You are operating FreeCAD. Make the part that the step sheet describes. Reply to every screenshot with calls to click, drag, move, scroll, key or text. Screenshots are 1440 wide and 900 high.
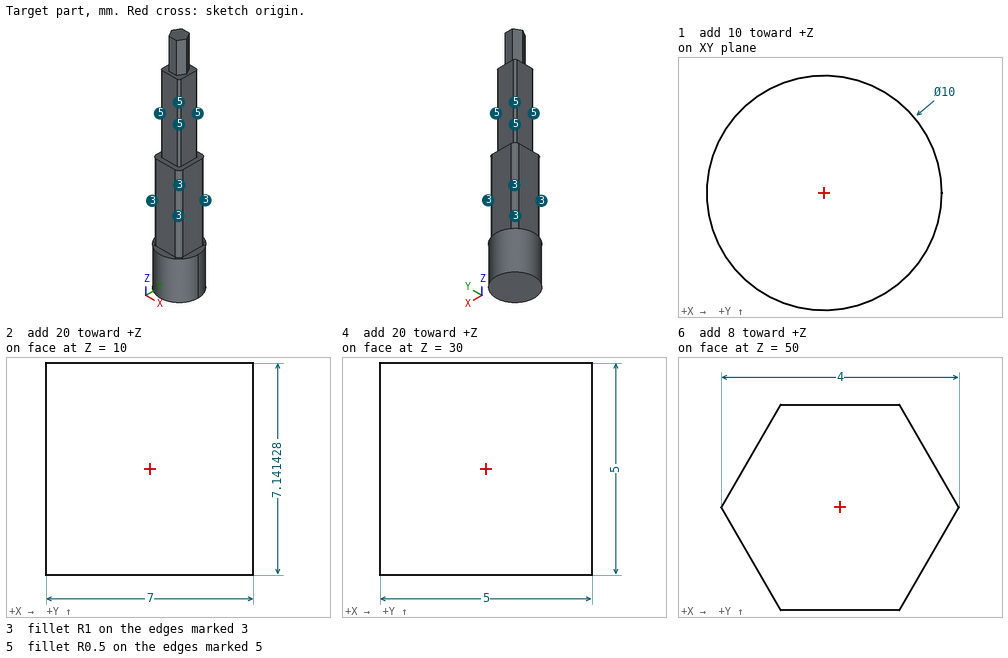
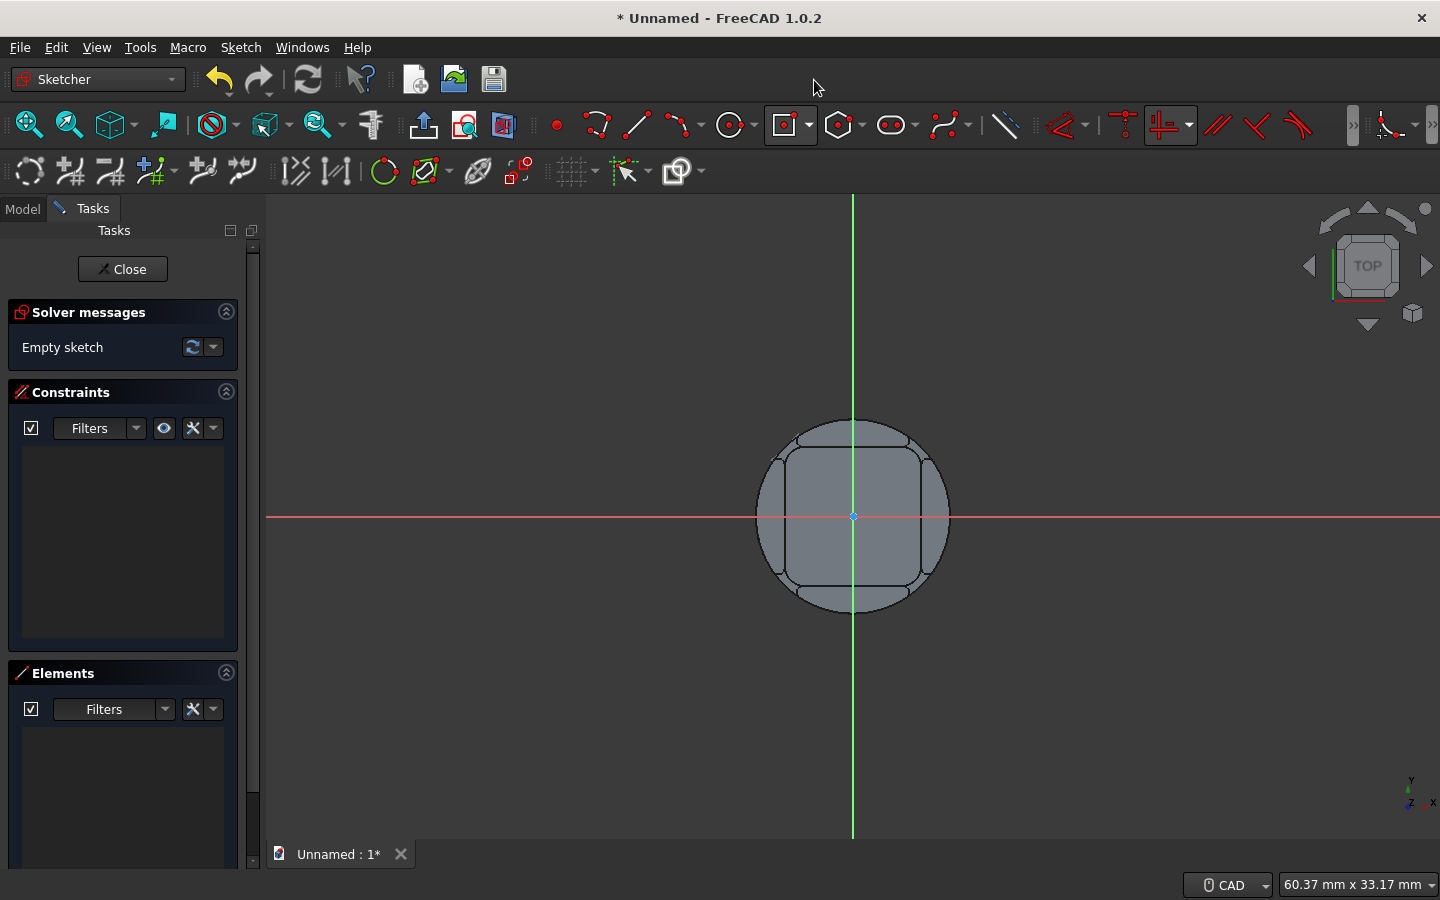
scroll(875, 516, up, 7)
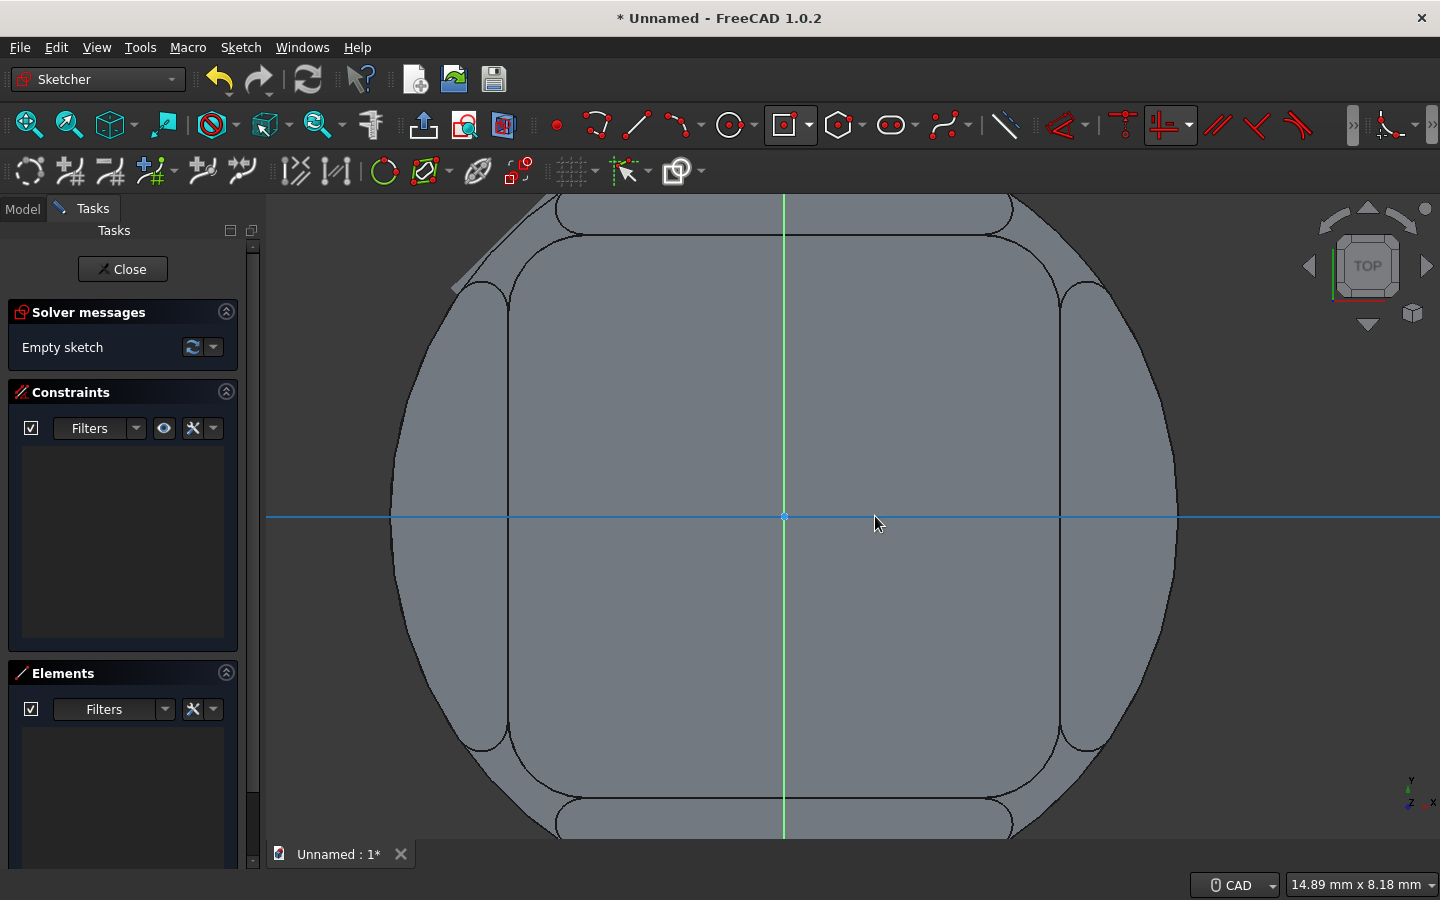
click(784, 126)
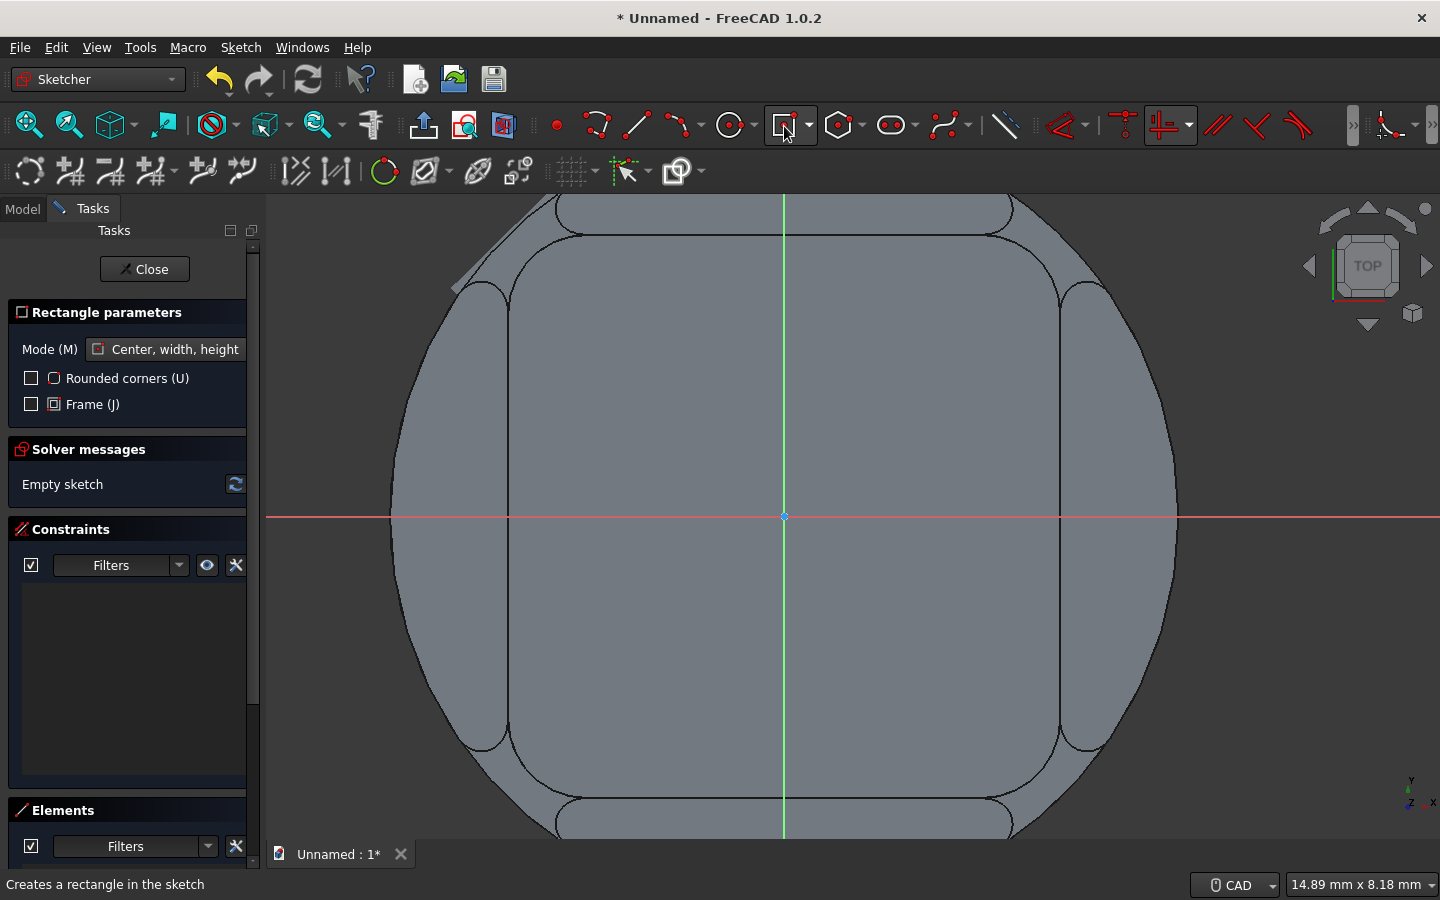
click(784, 516)
click(981, 319)
key(Escape)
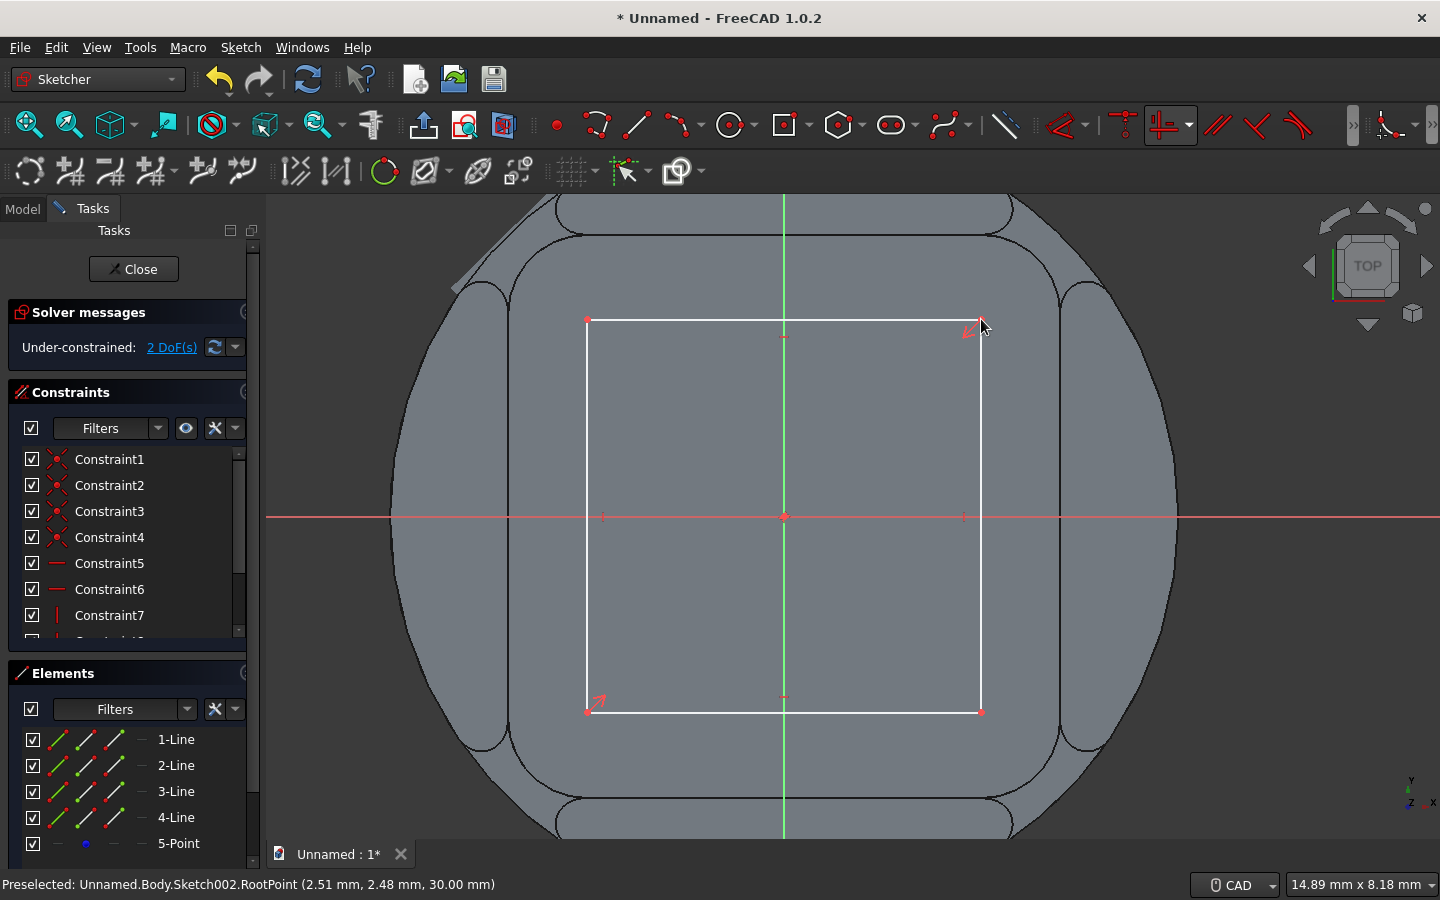
click(1060, 126)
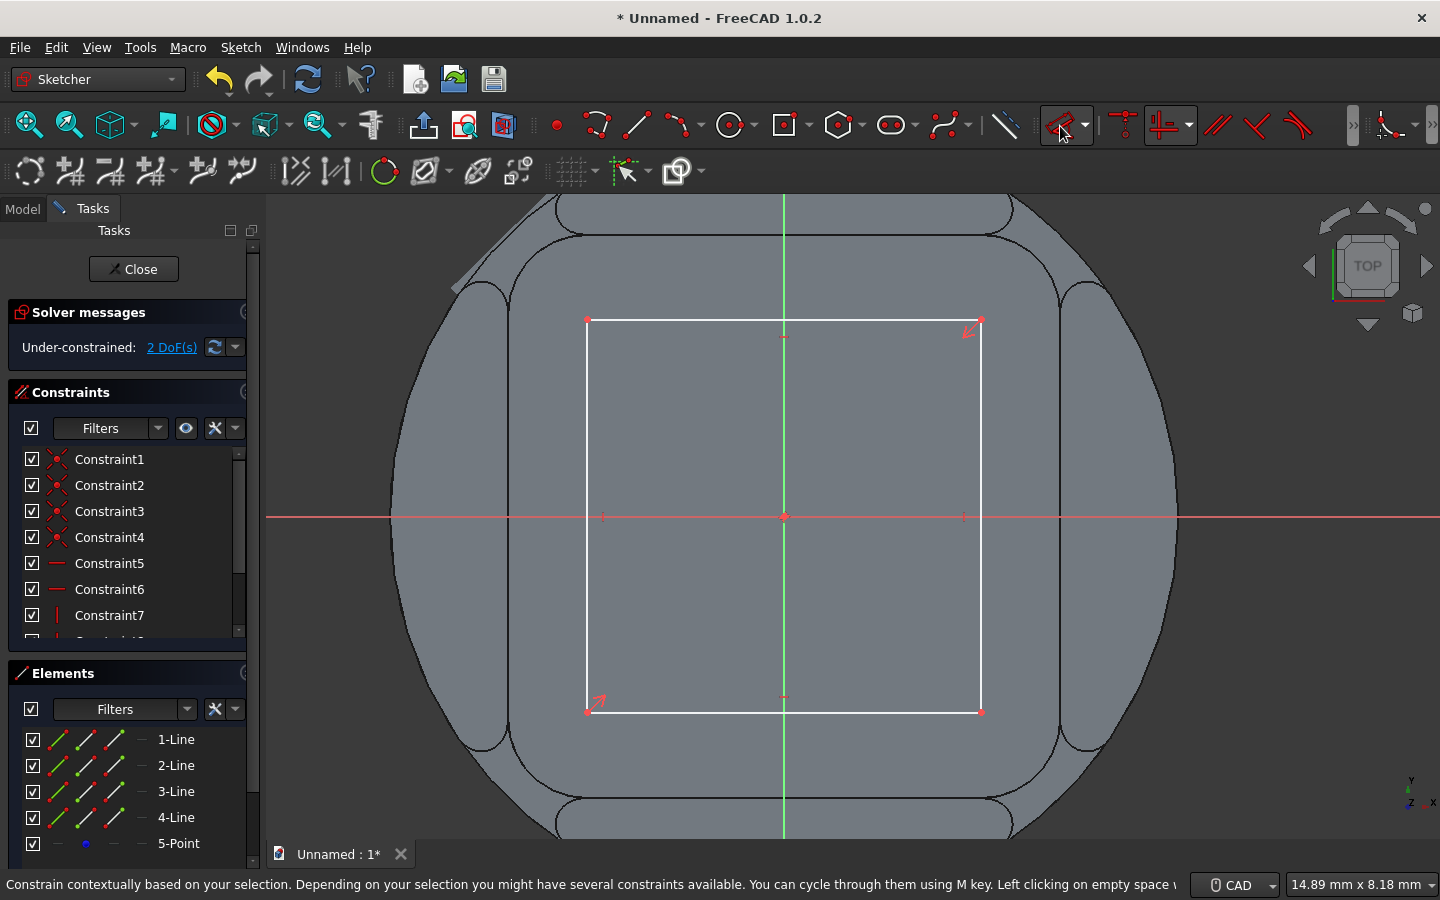
click(705, 713)
click(694, 747)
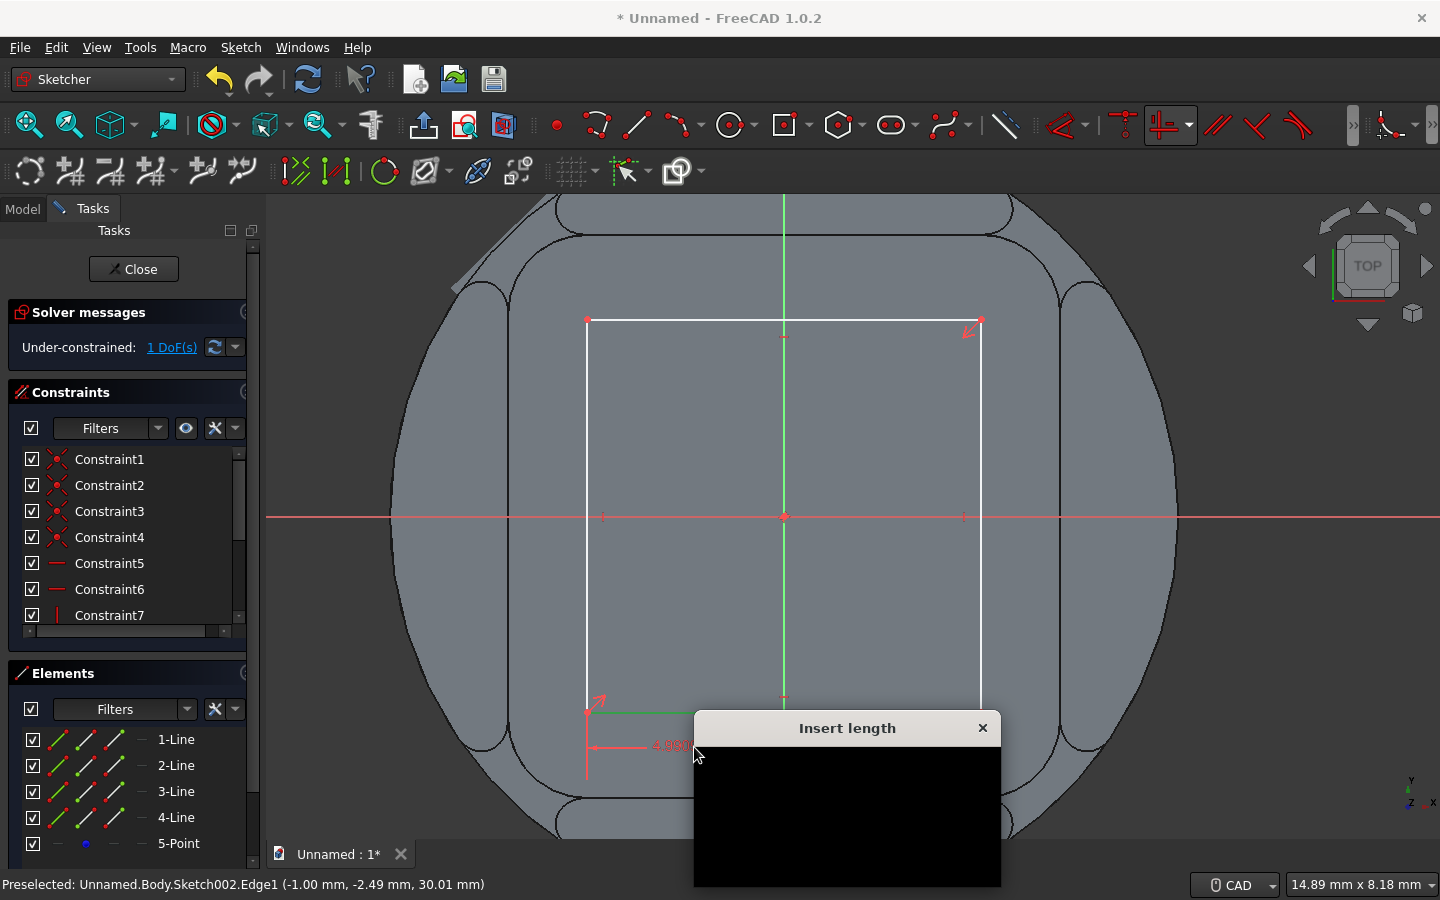
text(5)
key(Return)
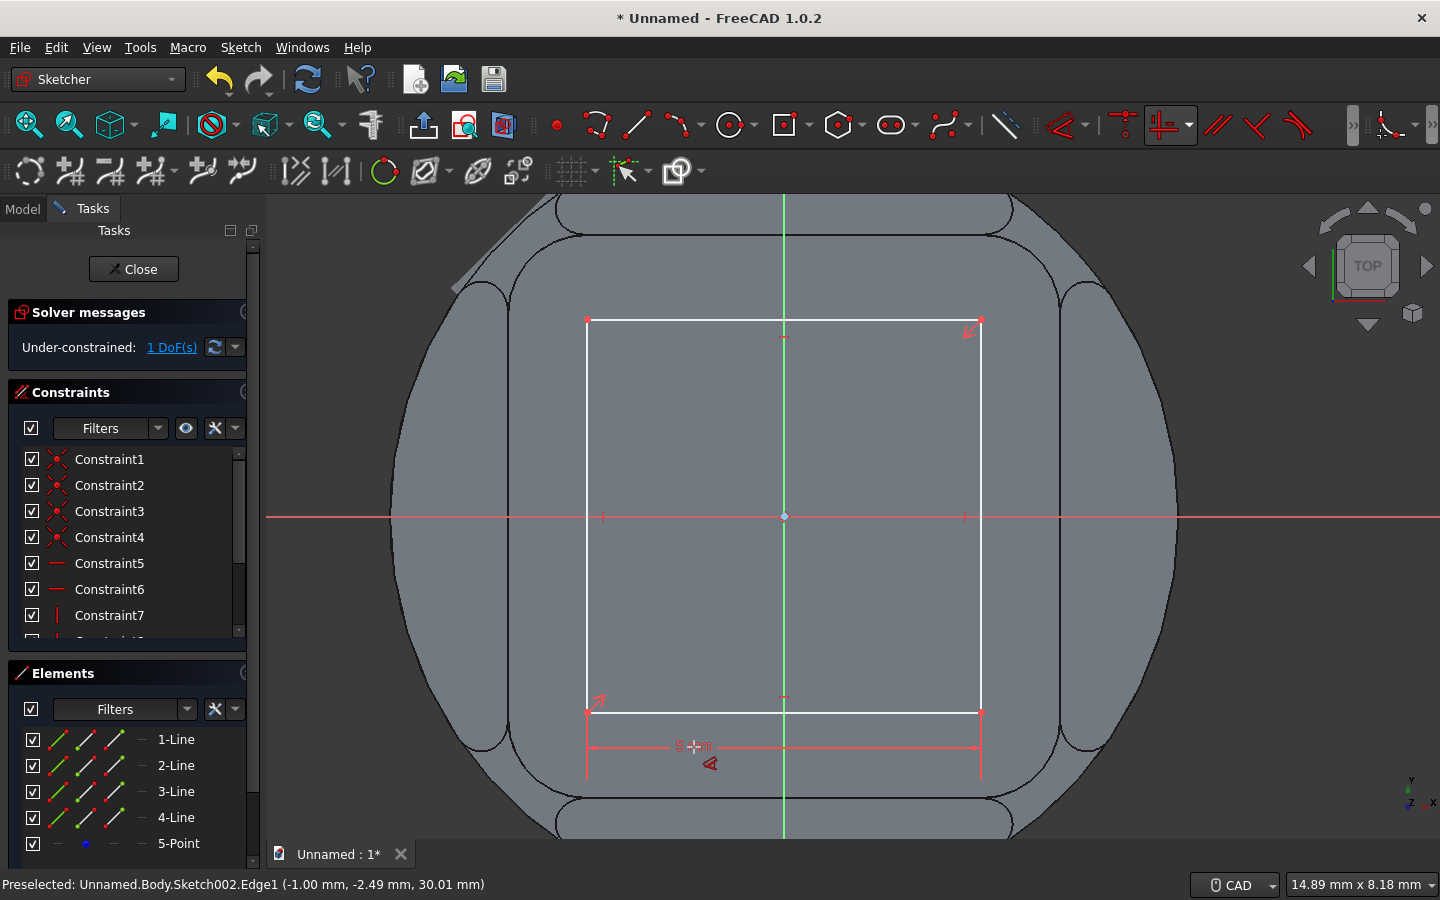
click(981, 595)
click(1015, 426)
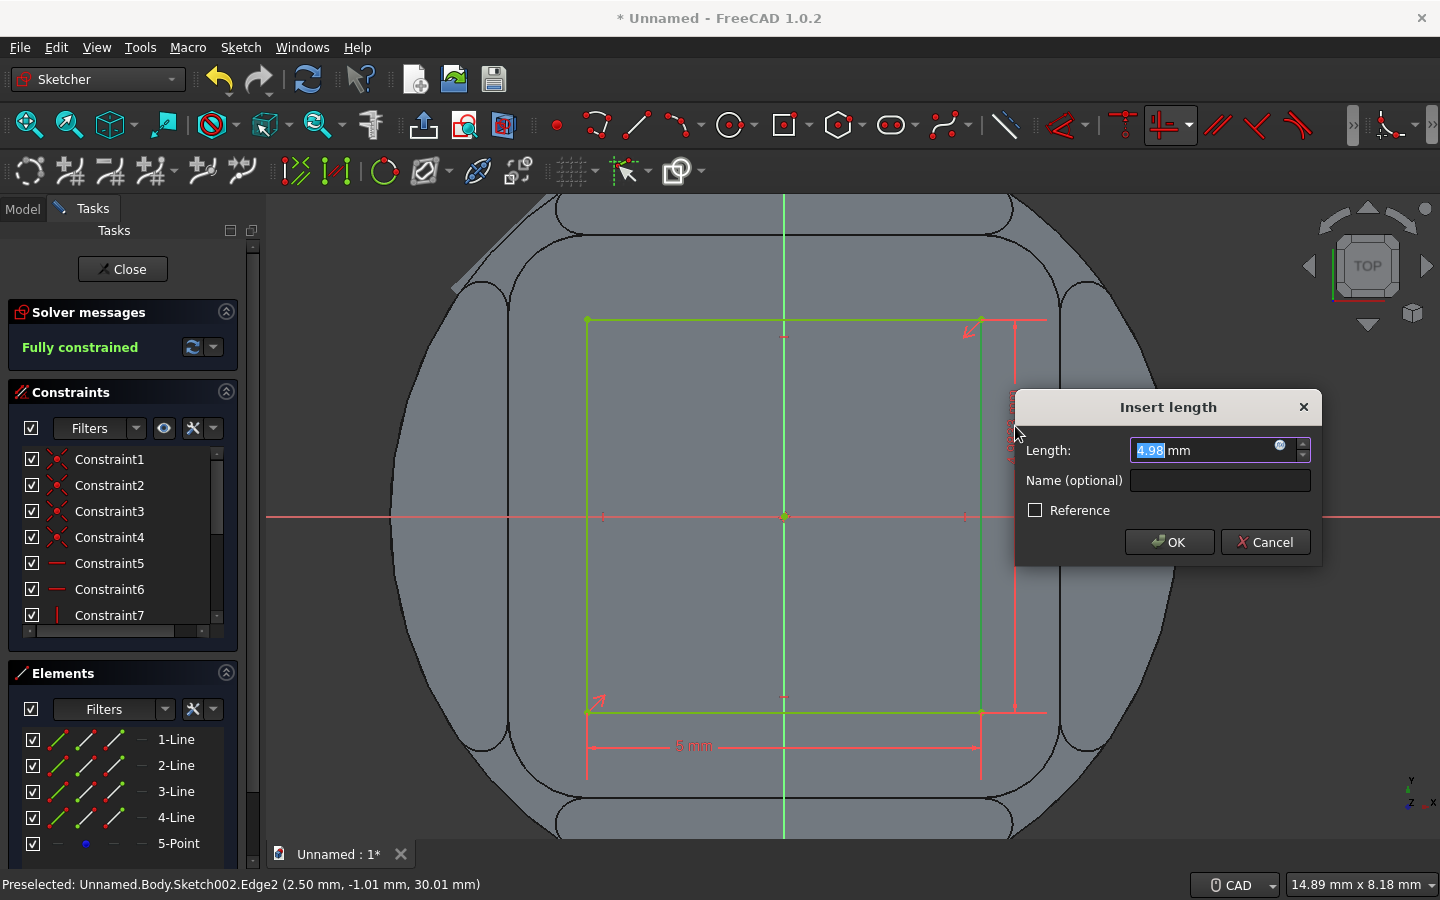
text(5)
key(Return)
key(Escape)